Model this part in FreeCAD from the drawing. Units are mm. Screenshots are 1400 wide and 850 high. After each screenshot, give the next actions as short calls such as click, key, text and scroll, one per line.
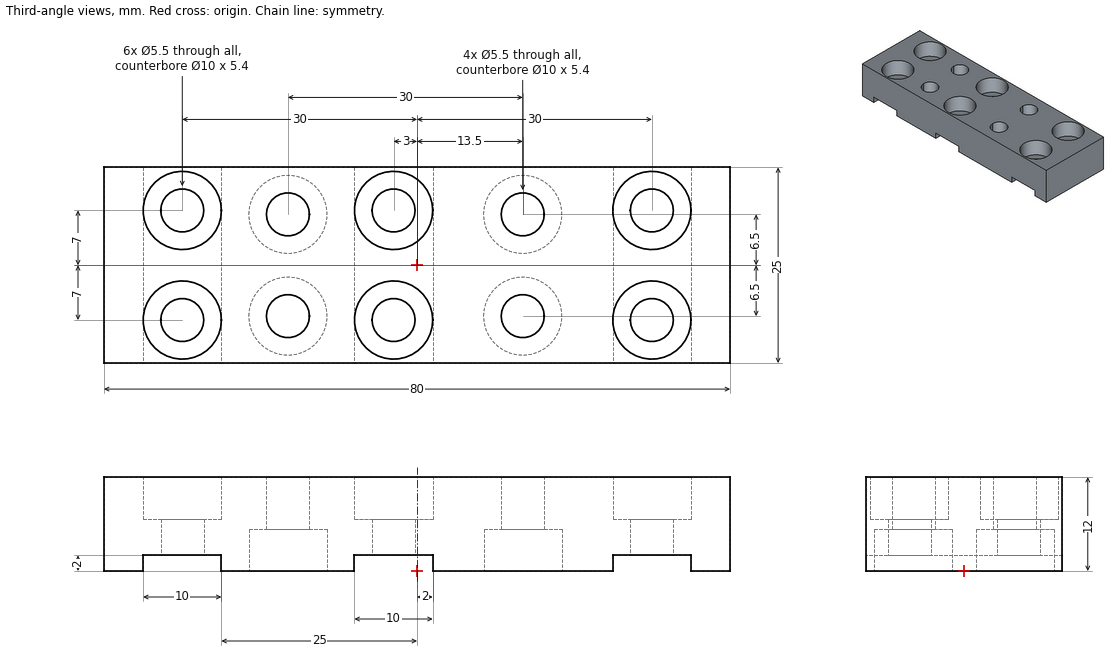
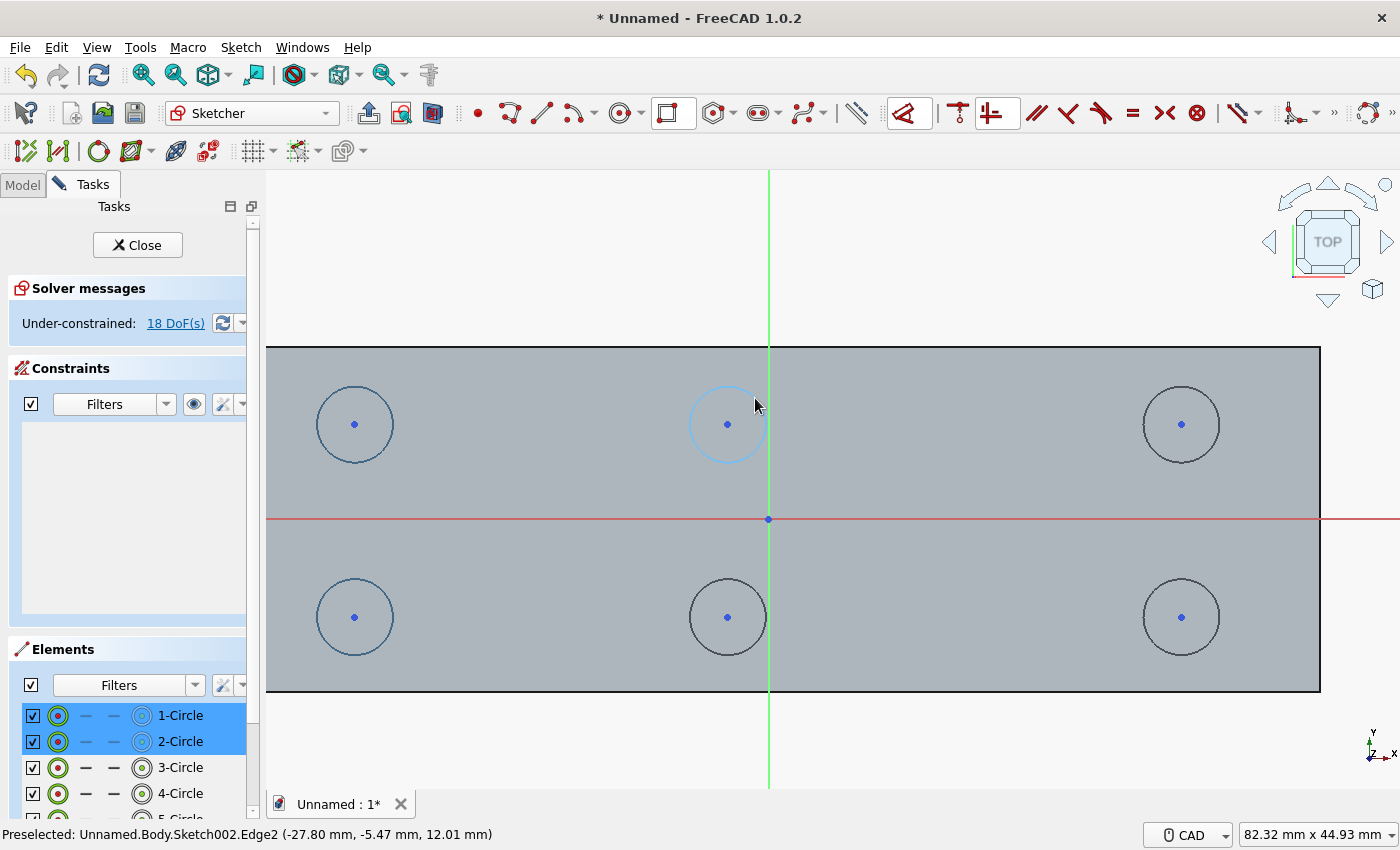
click(755, 398)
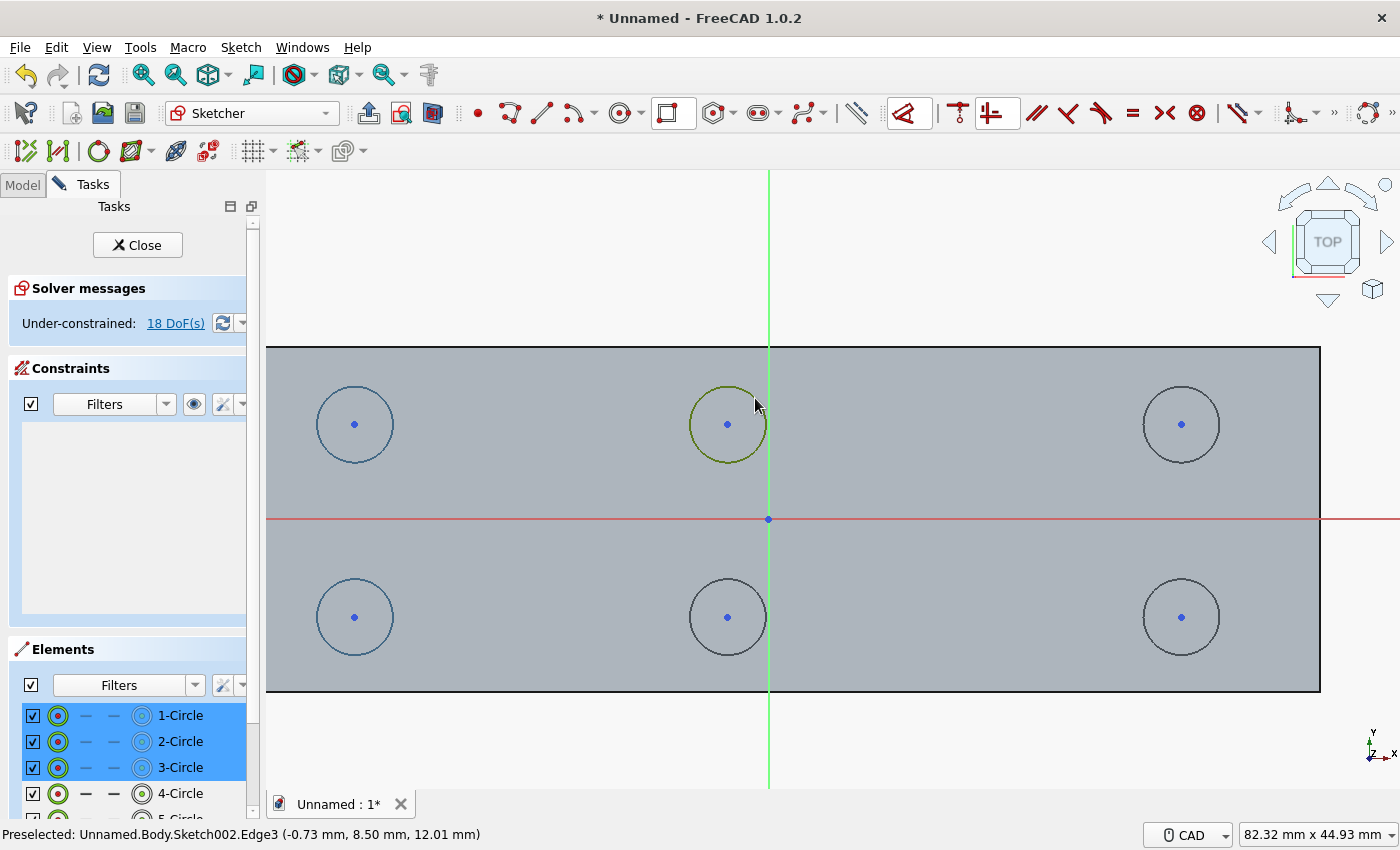
click(755, 590)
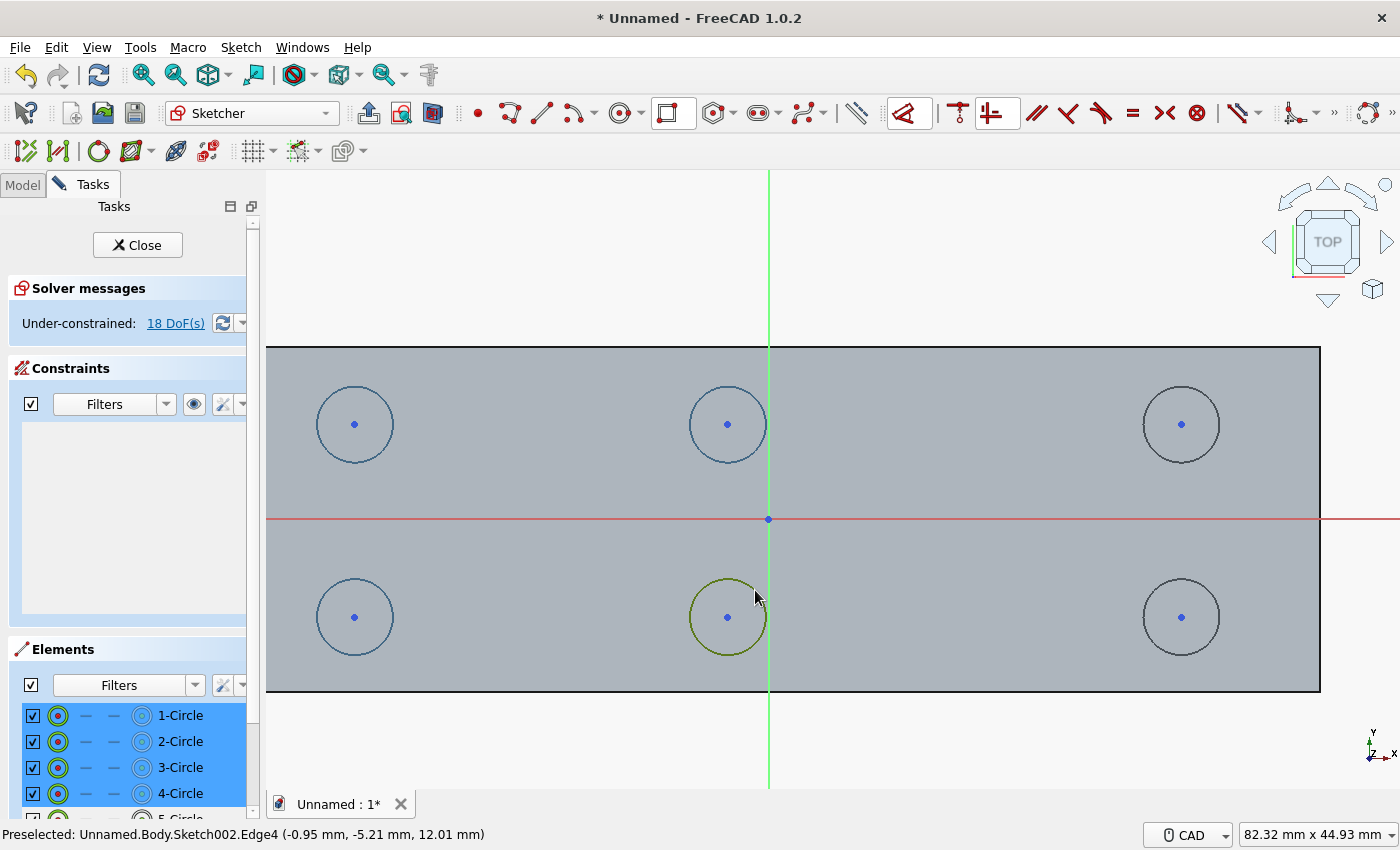
click(1208, 398)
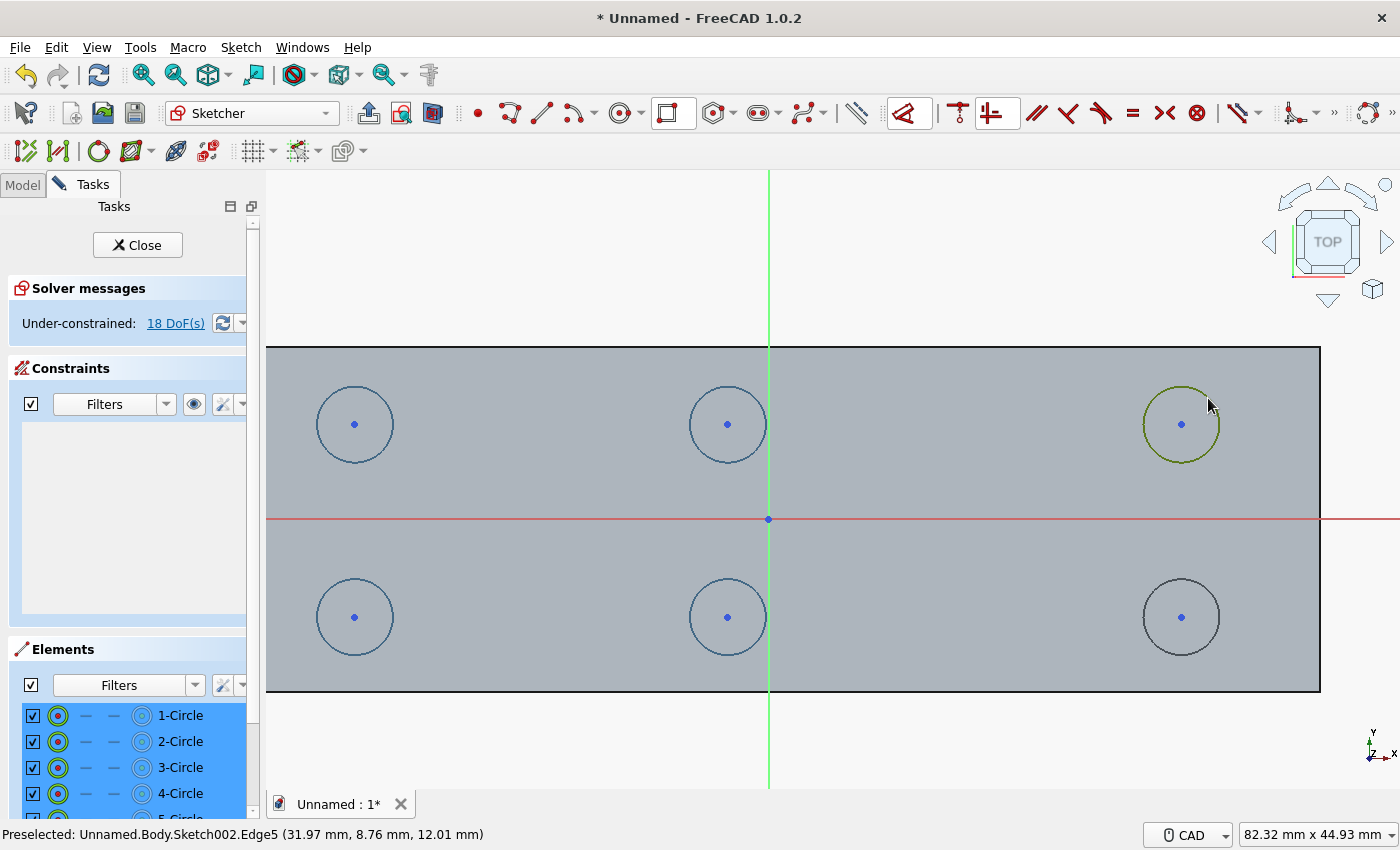
click(1208, 590)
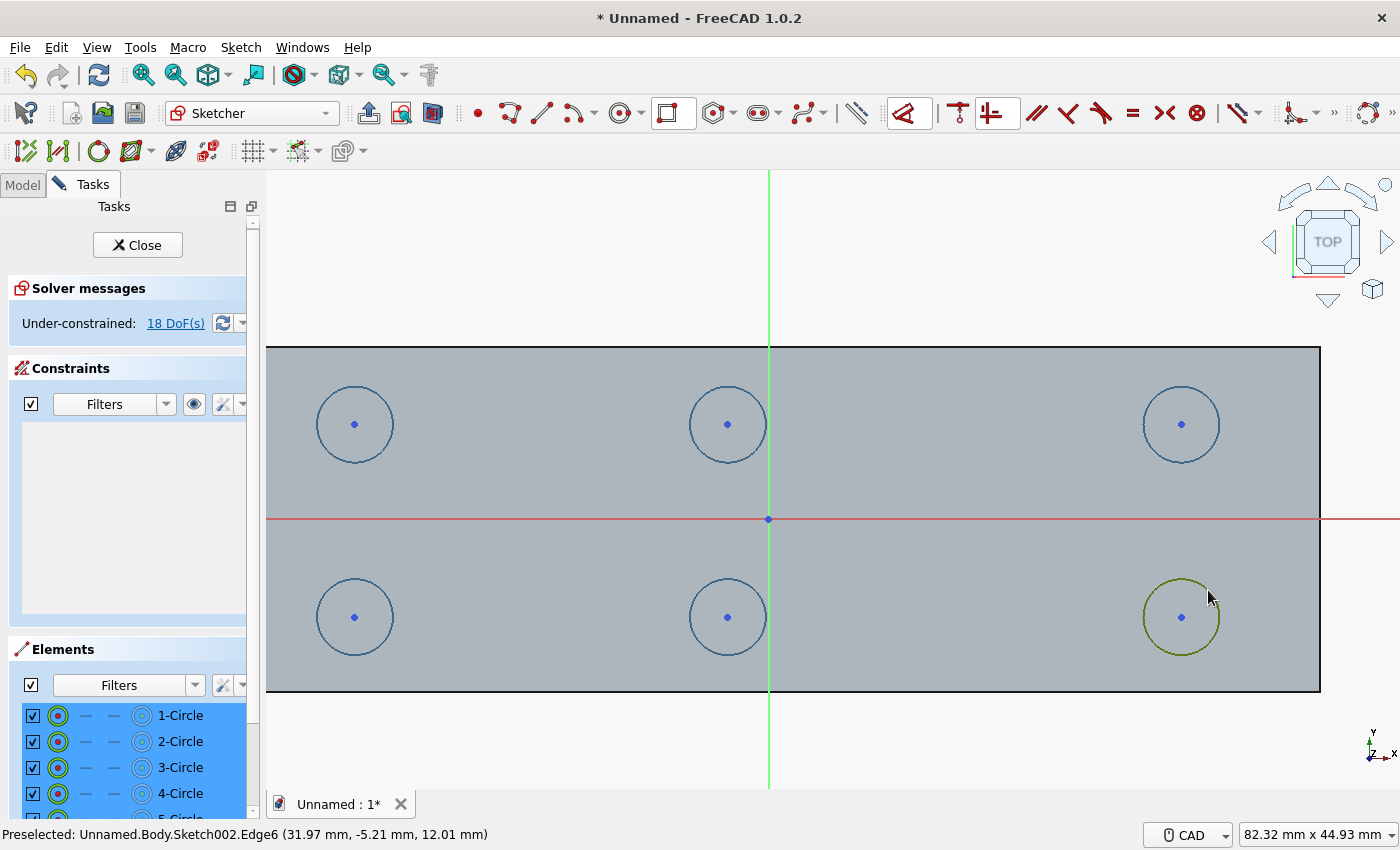
click(1134, 114)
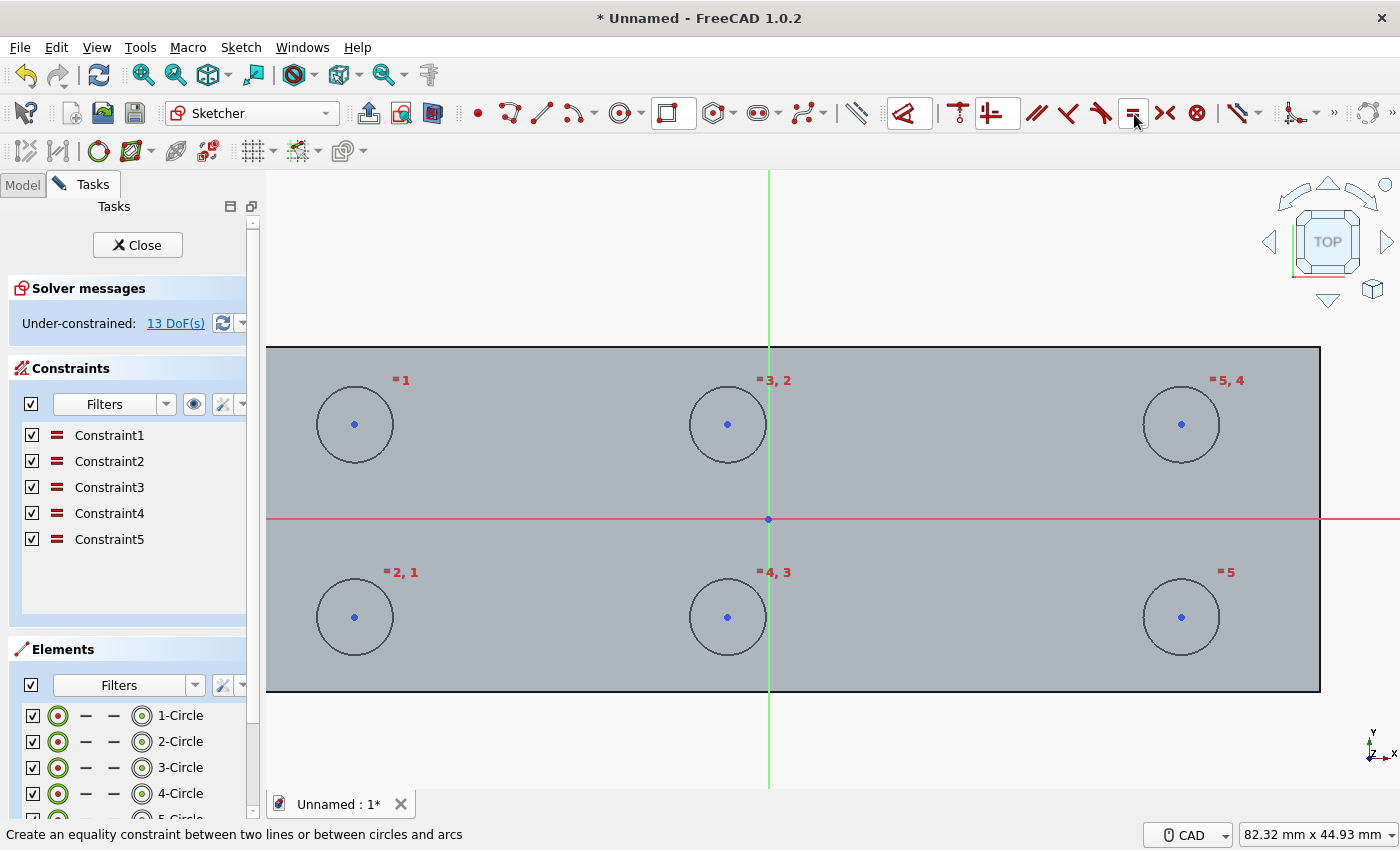
click(355, 425)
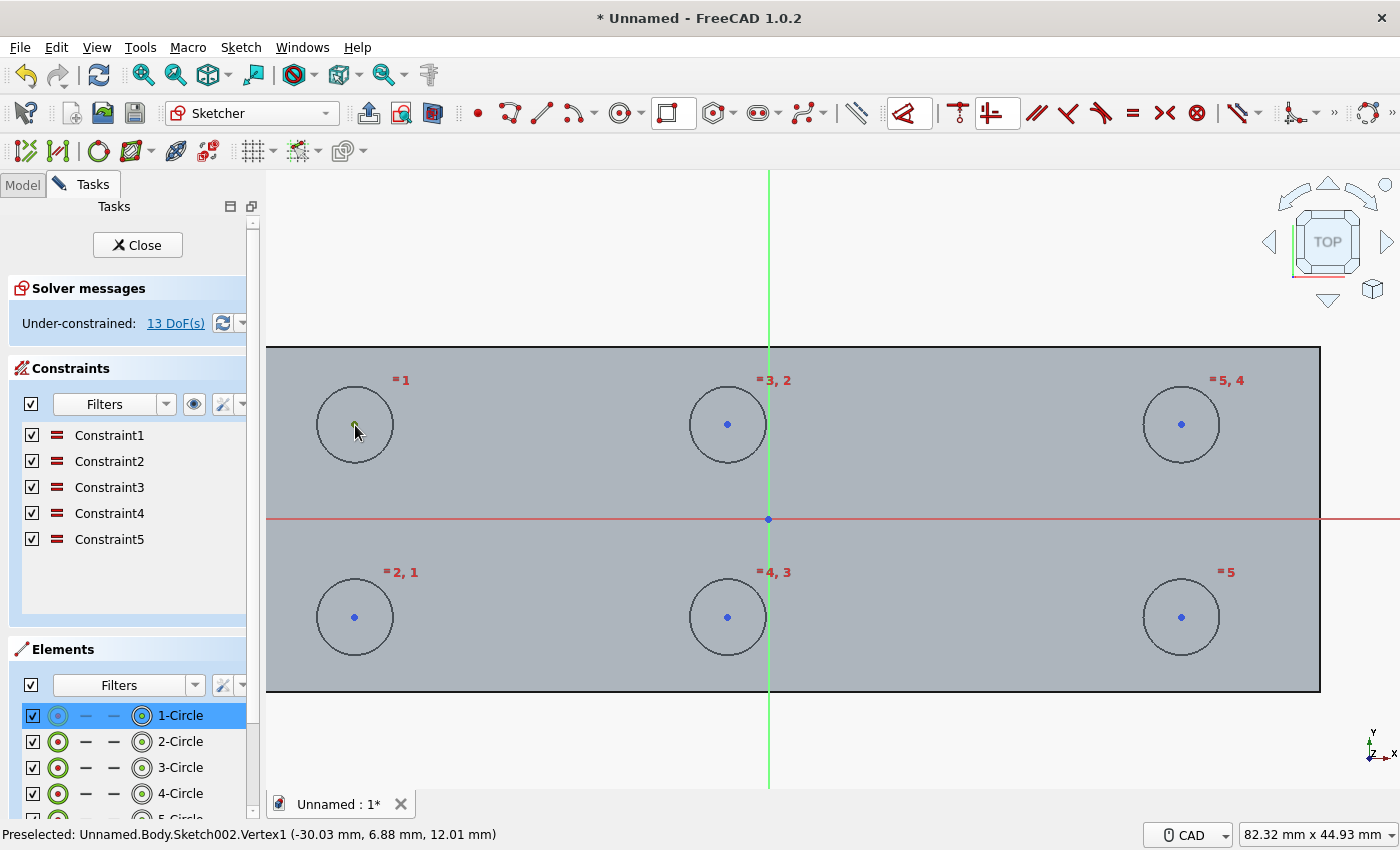
click(355, 617)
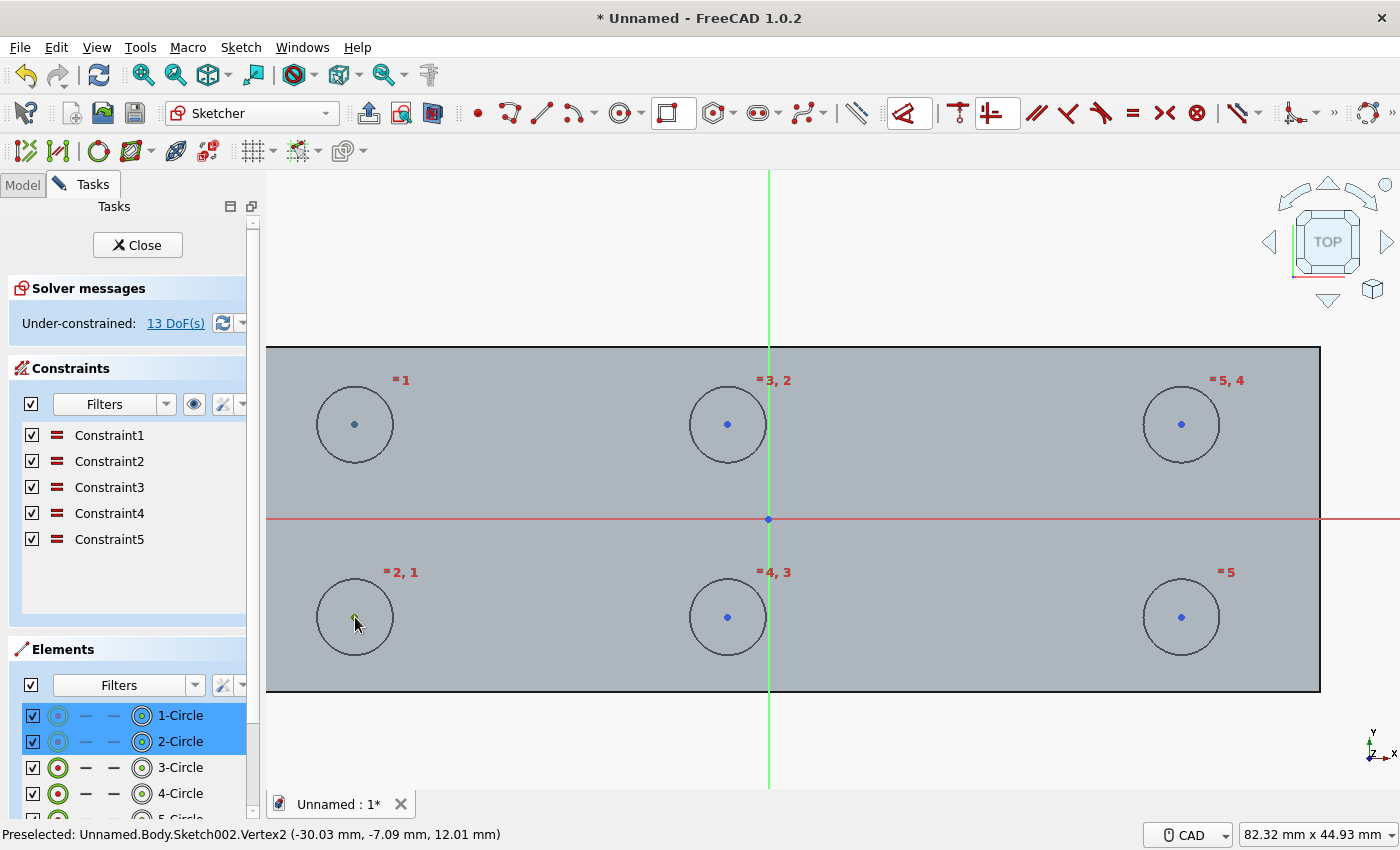
click(1014, 114)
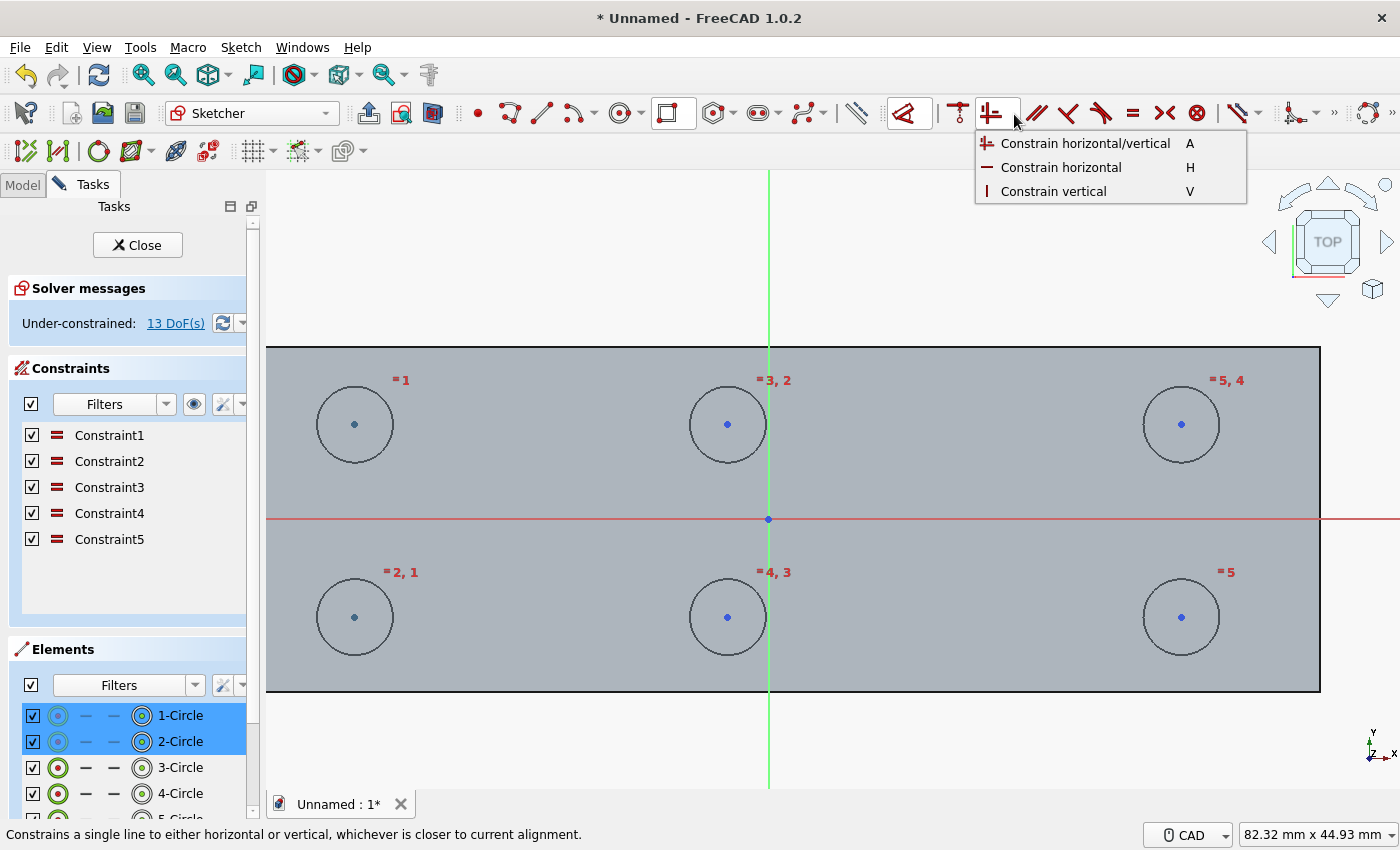
click(1111, 191)